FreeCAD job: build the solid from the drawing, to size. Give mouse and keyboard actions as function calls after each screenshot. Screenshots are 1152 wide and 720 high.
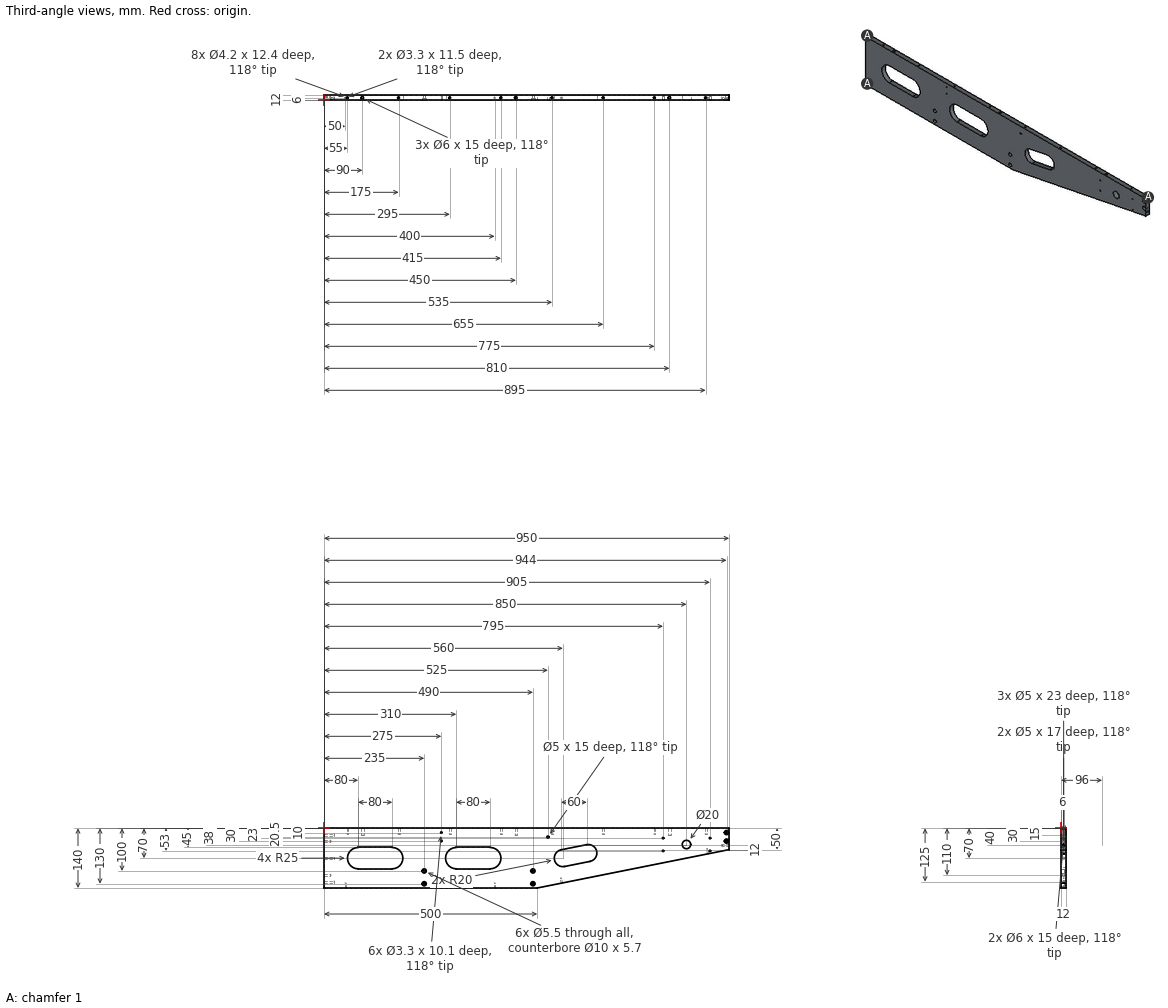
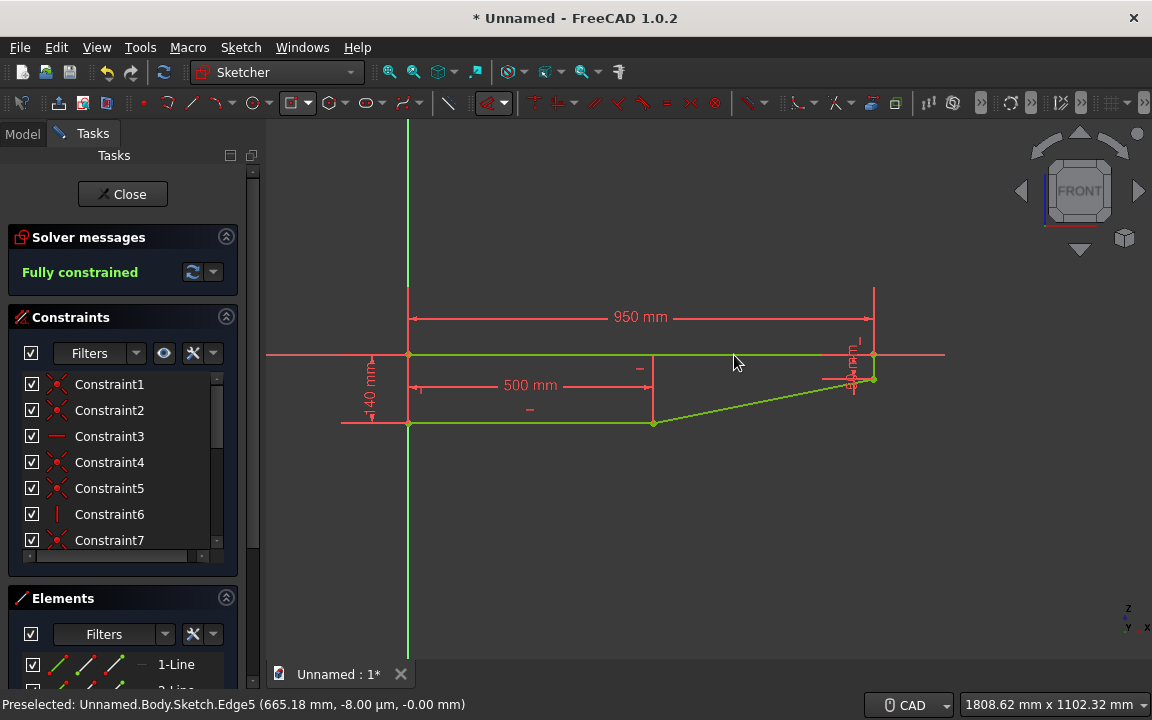
click(123, 194)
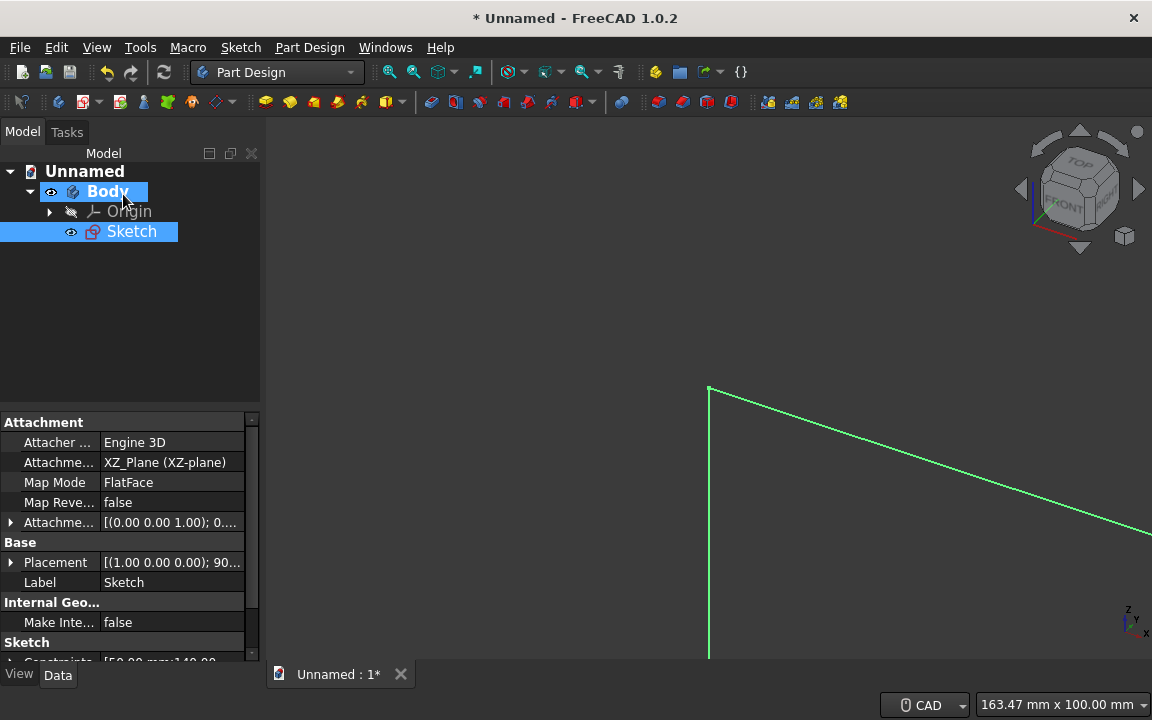
click(266, 102)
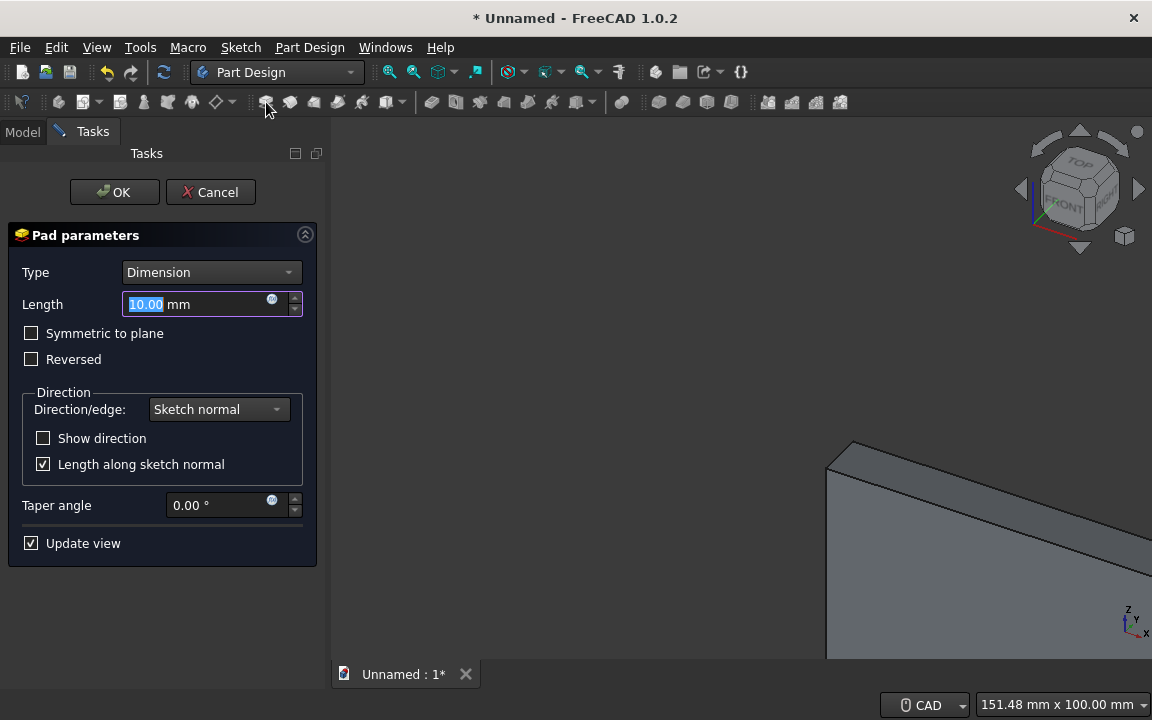
text(12)
key(Tab)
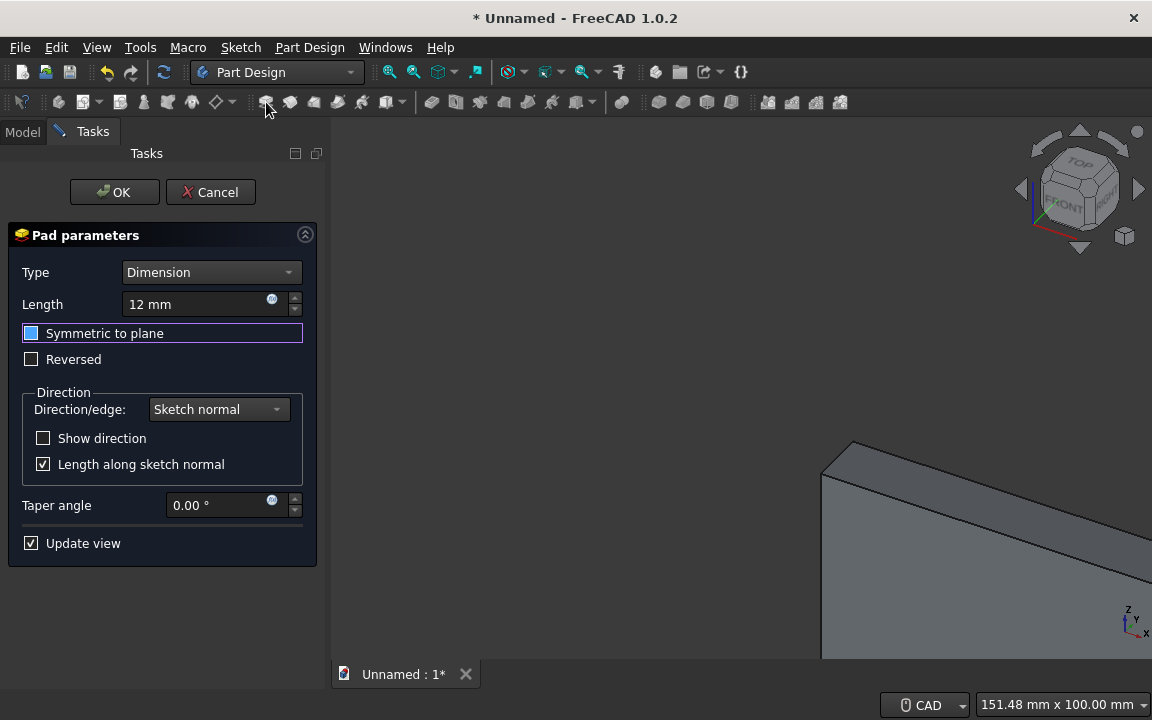
click(30, 359)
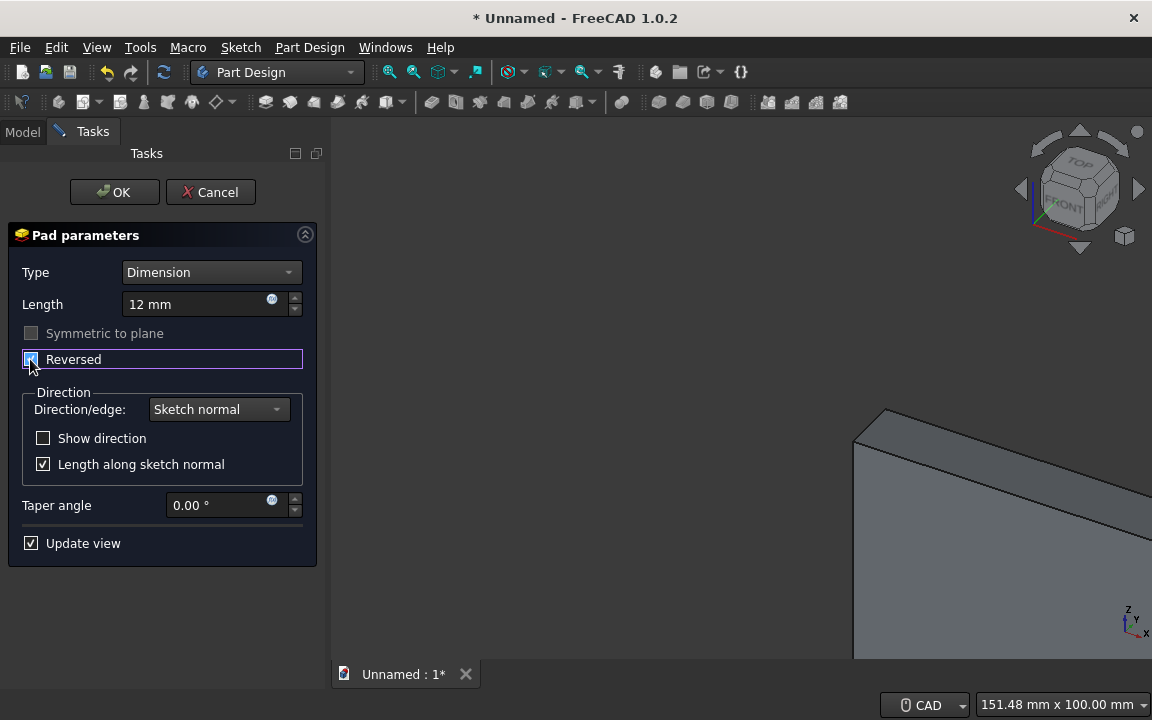
click(115, 192)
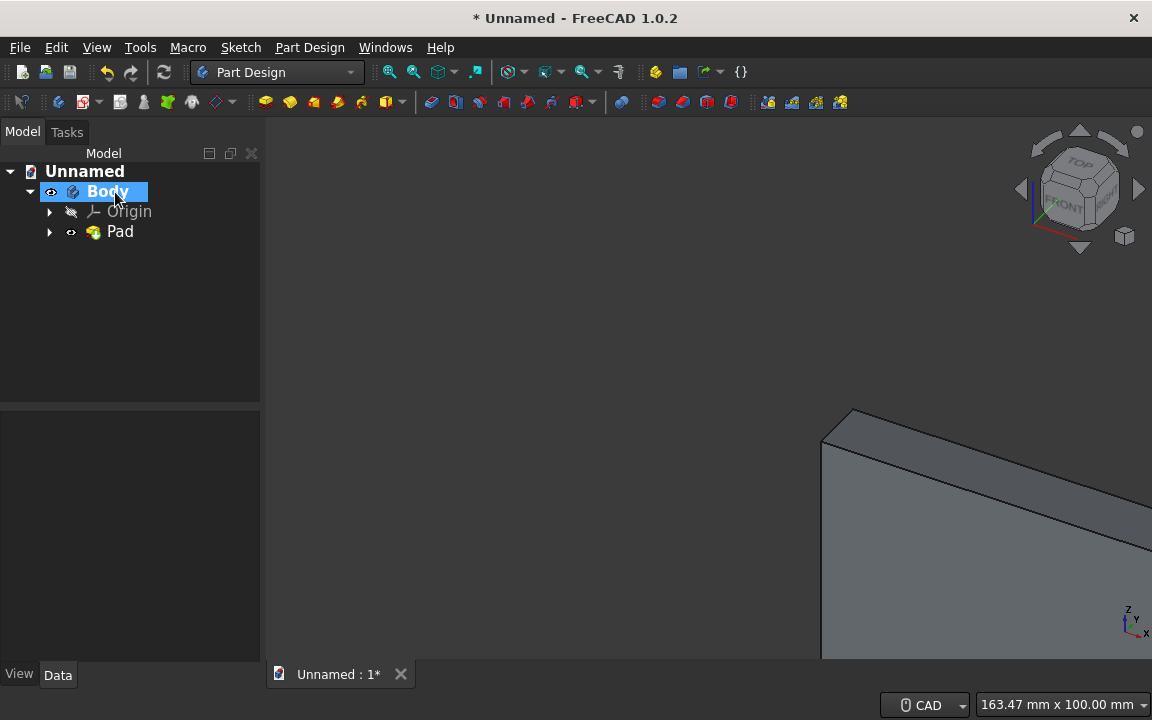
key(v)
key(f)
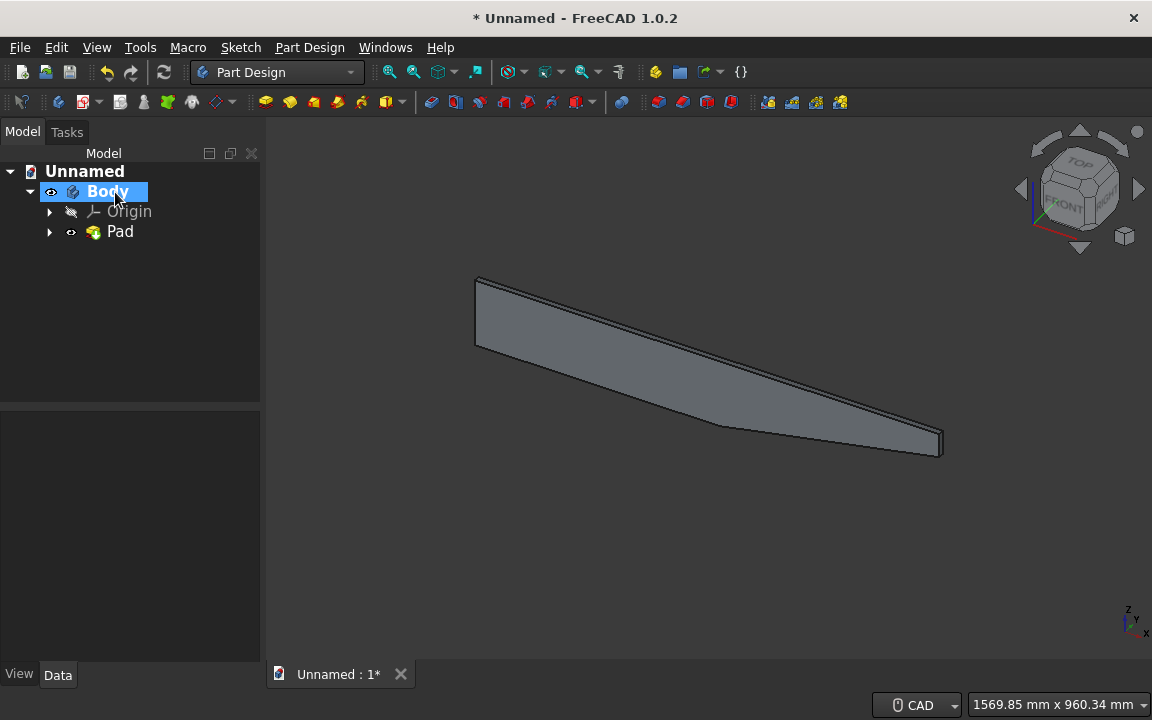
click(707, 389)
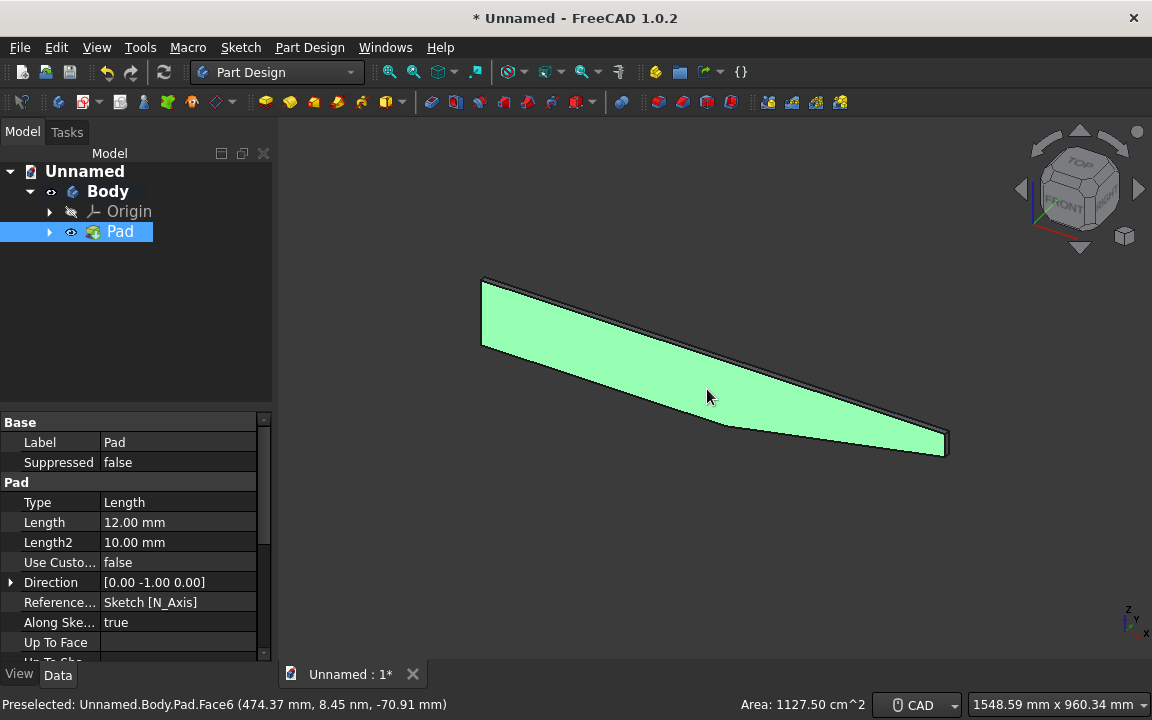
click(84, 102)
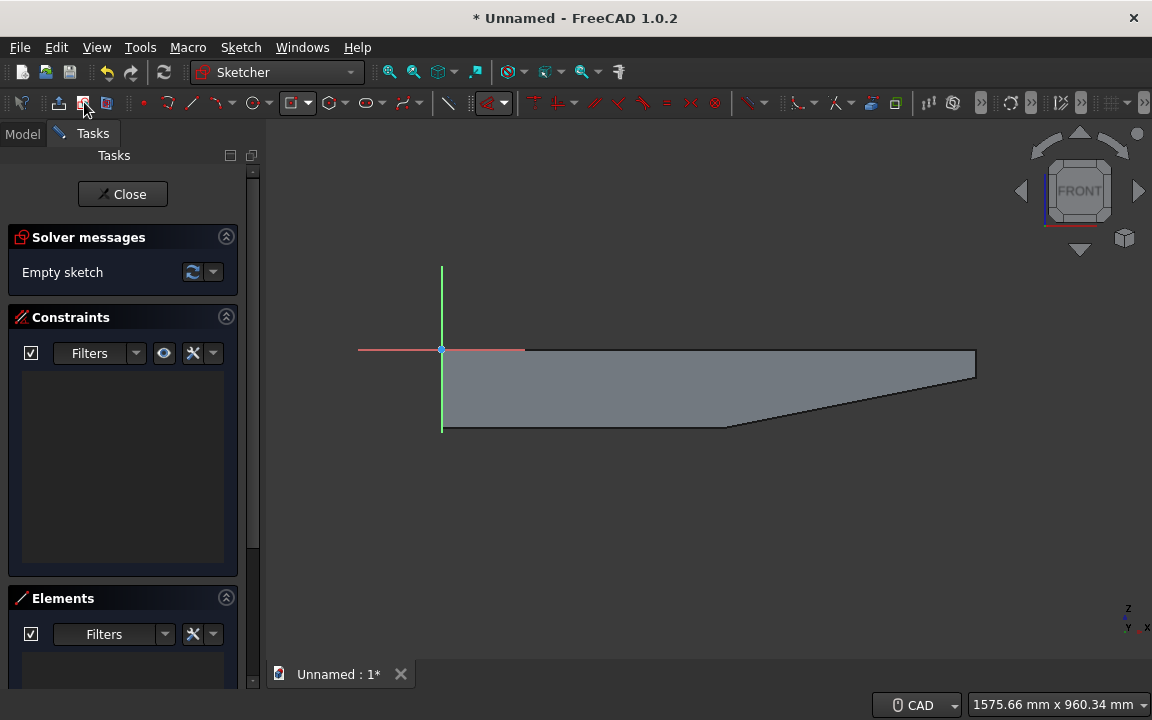
key(g)
key(s)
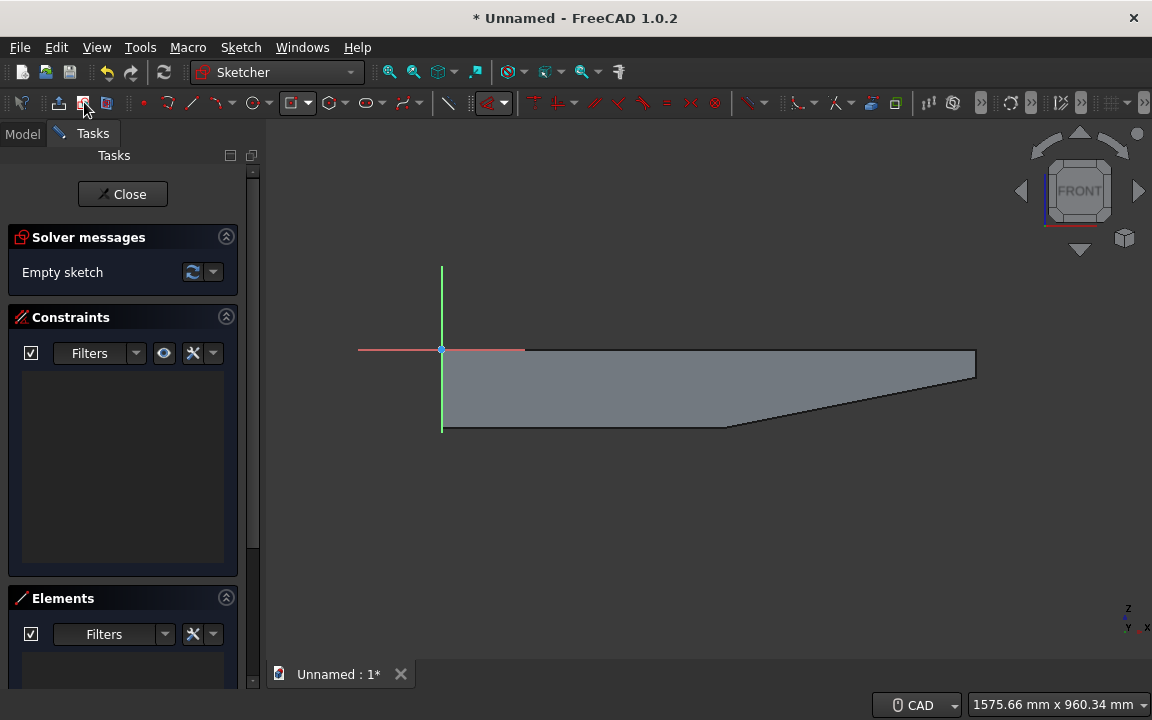
scroll(487, 389, up, 3)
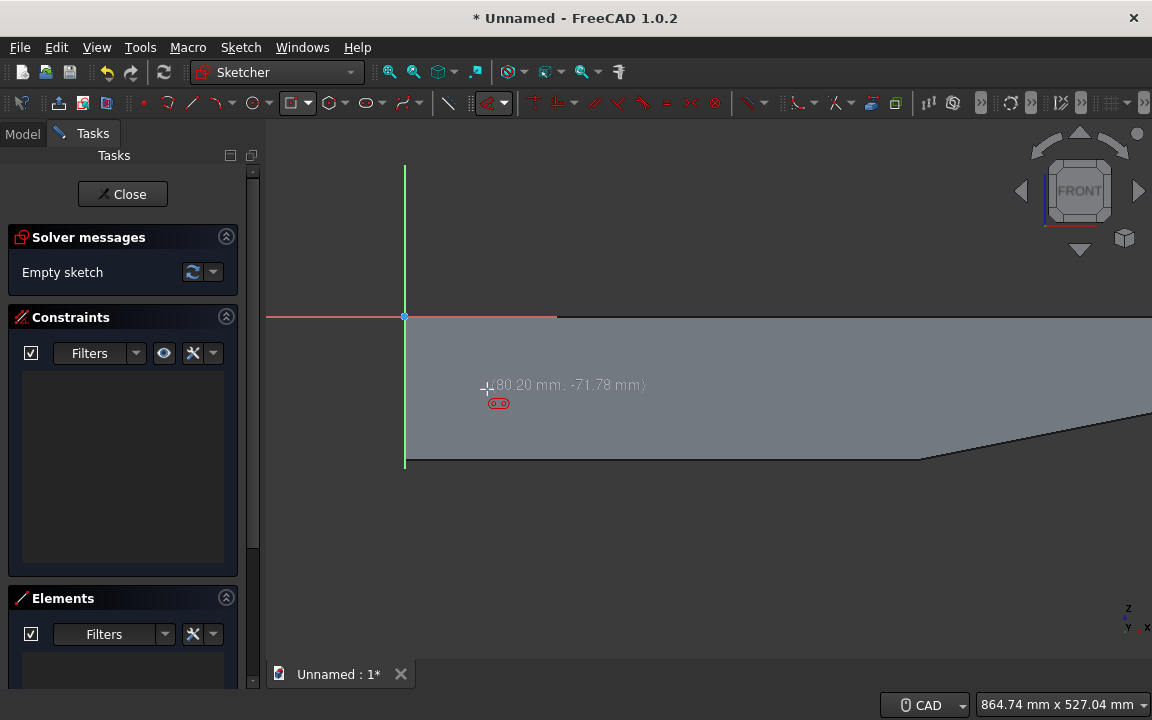
click(487, 389)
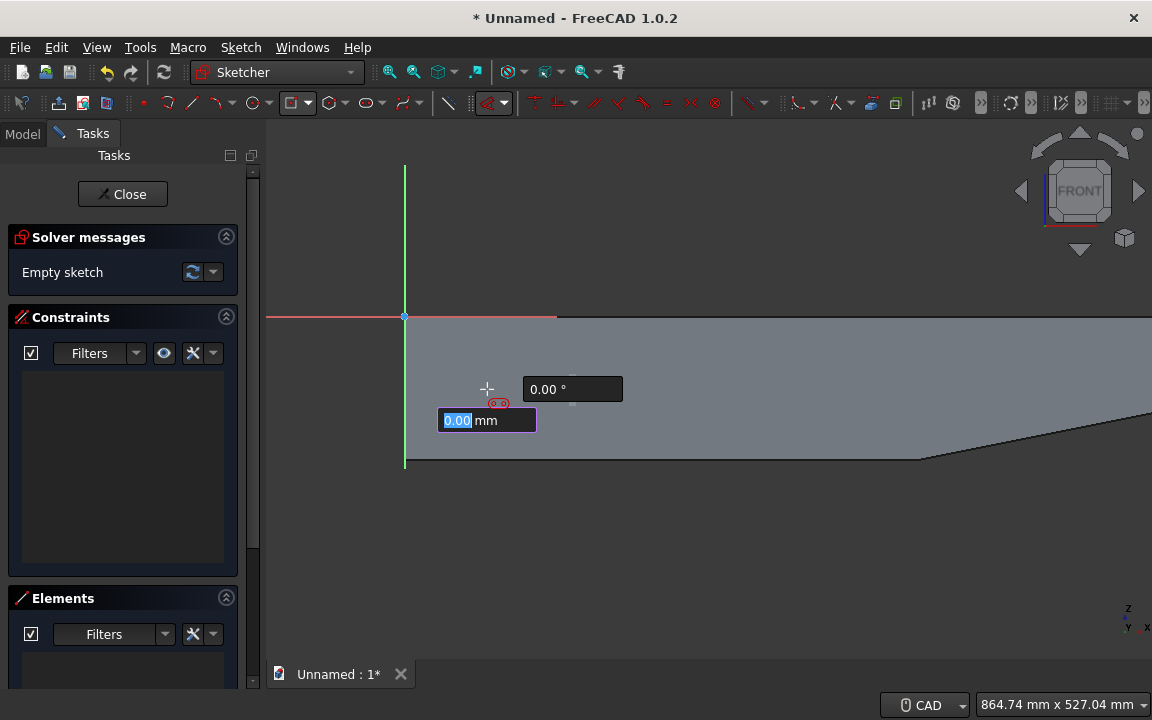
click(569, 389)